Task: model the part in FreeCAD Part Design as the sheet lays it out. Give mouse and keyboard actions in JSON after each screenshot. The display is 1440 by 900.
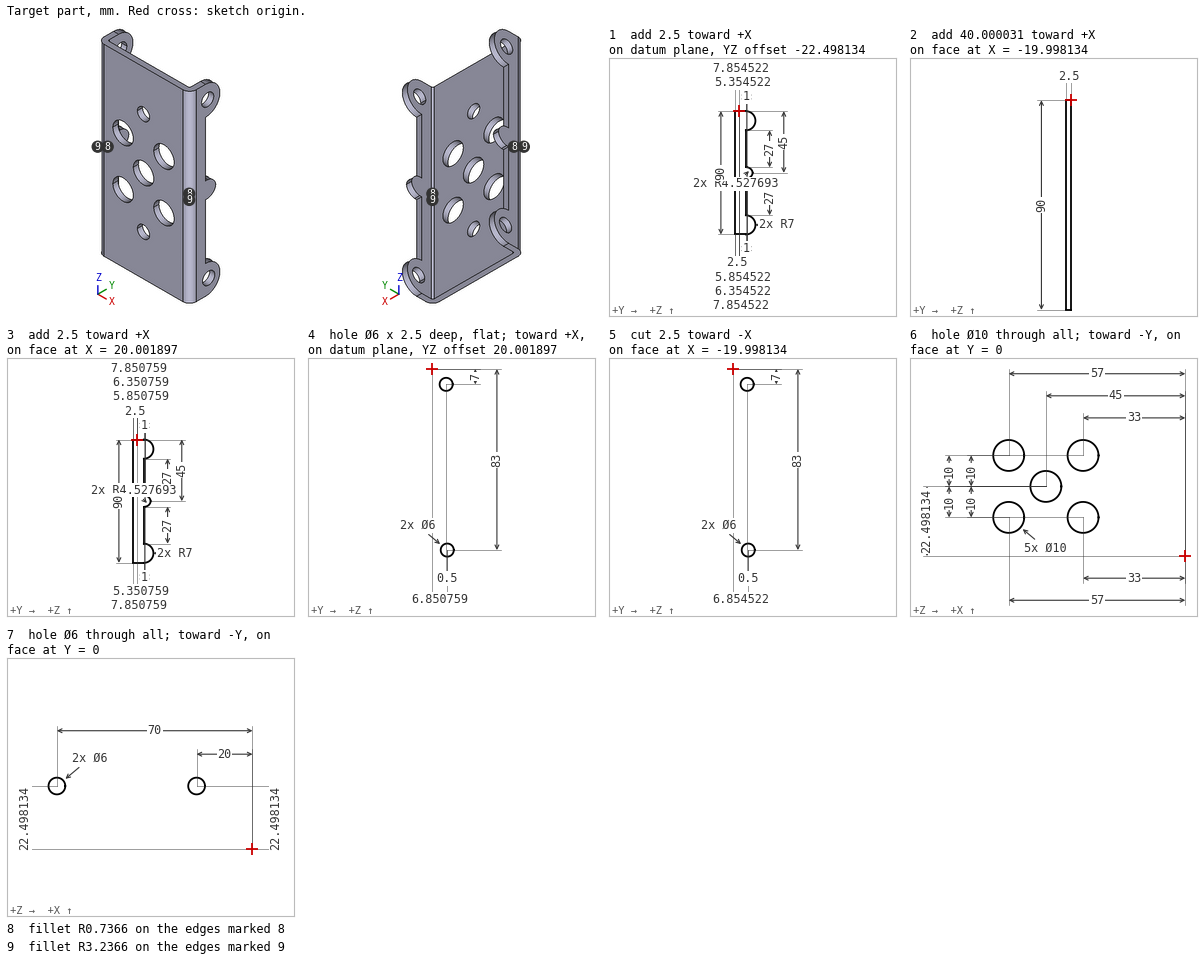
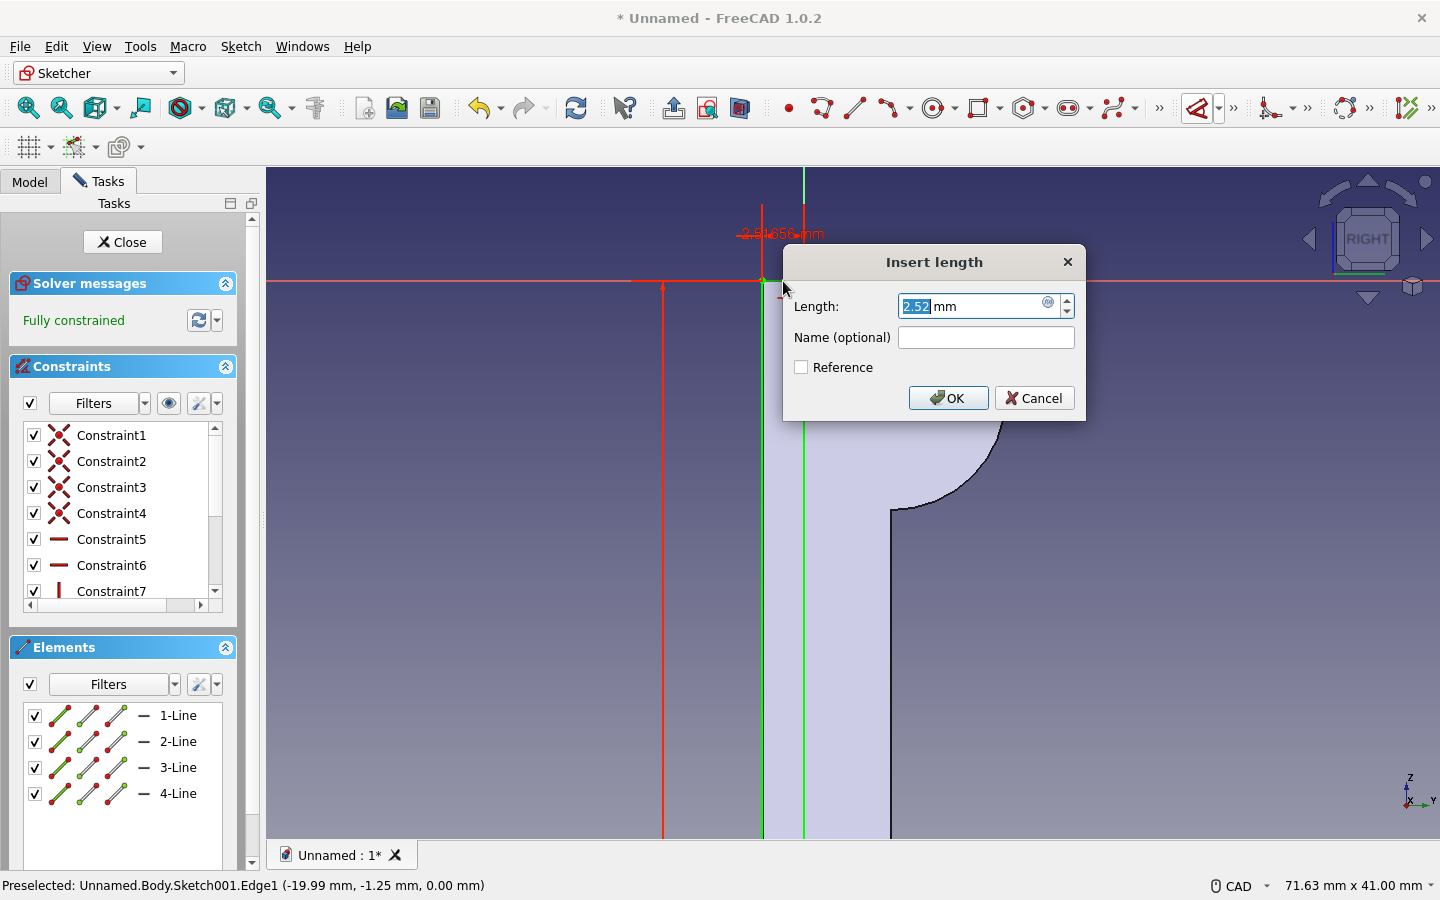
{"action": "type", "text": "2.5"}
{"action": "key", "text": "Return"}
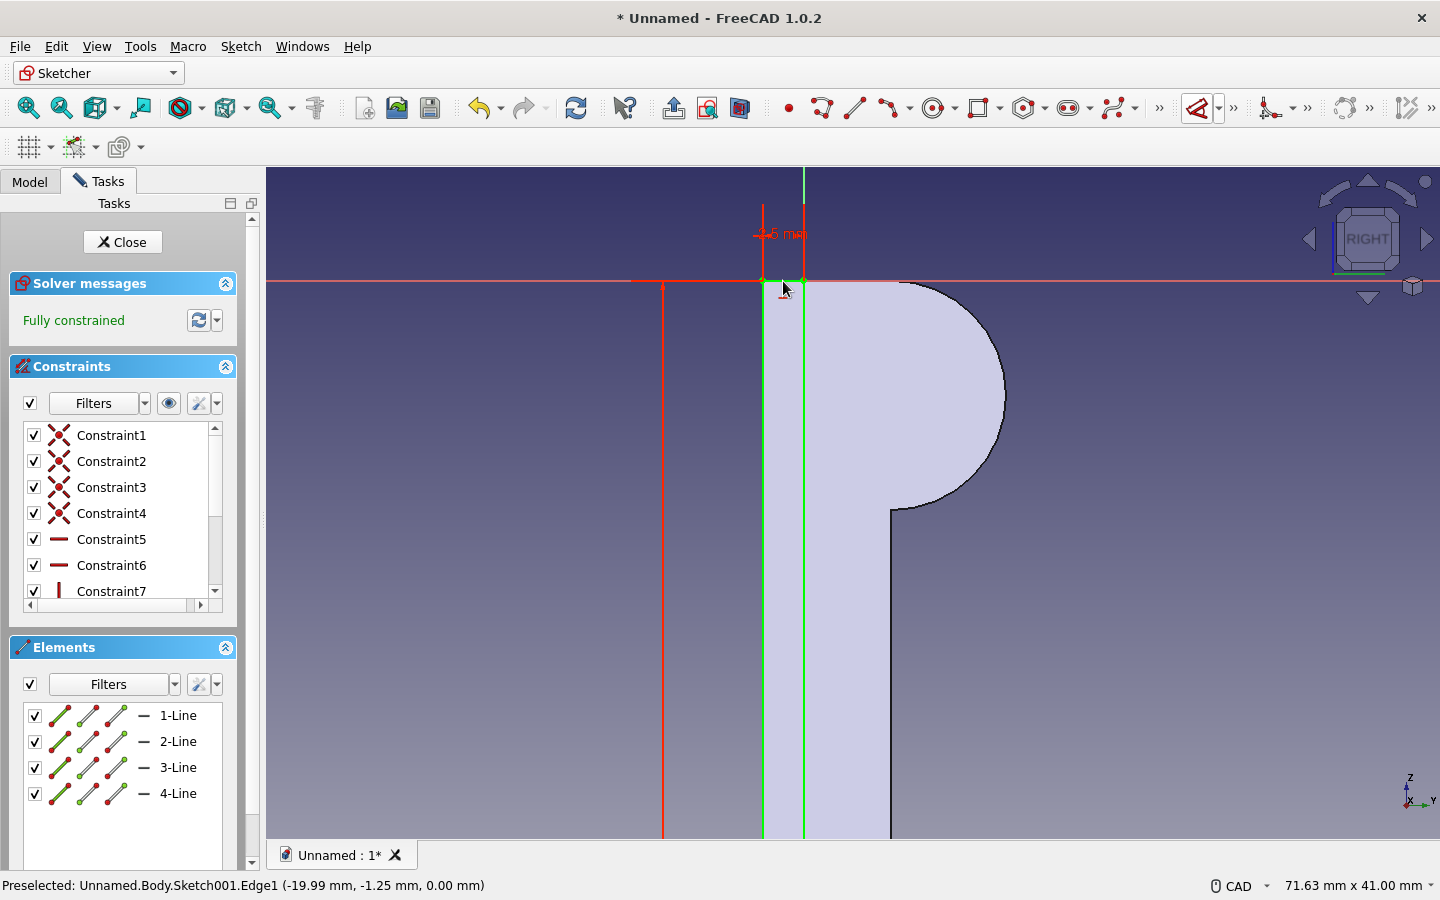
{"action": "left_click", "coordinate": [123, 242]}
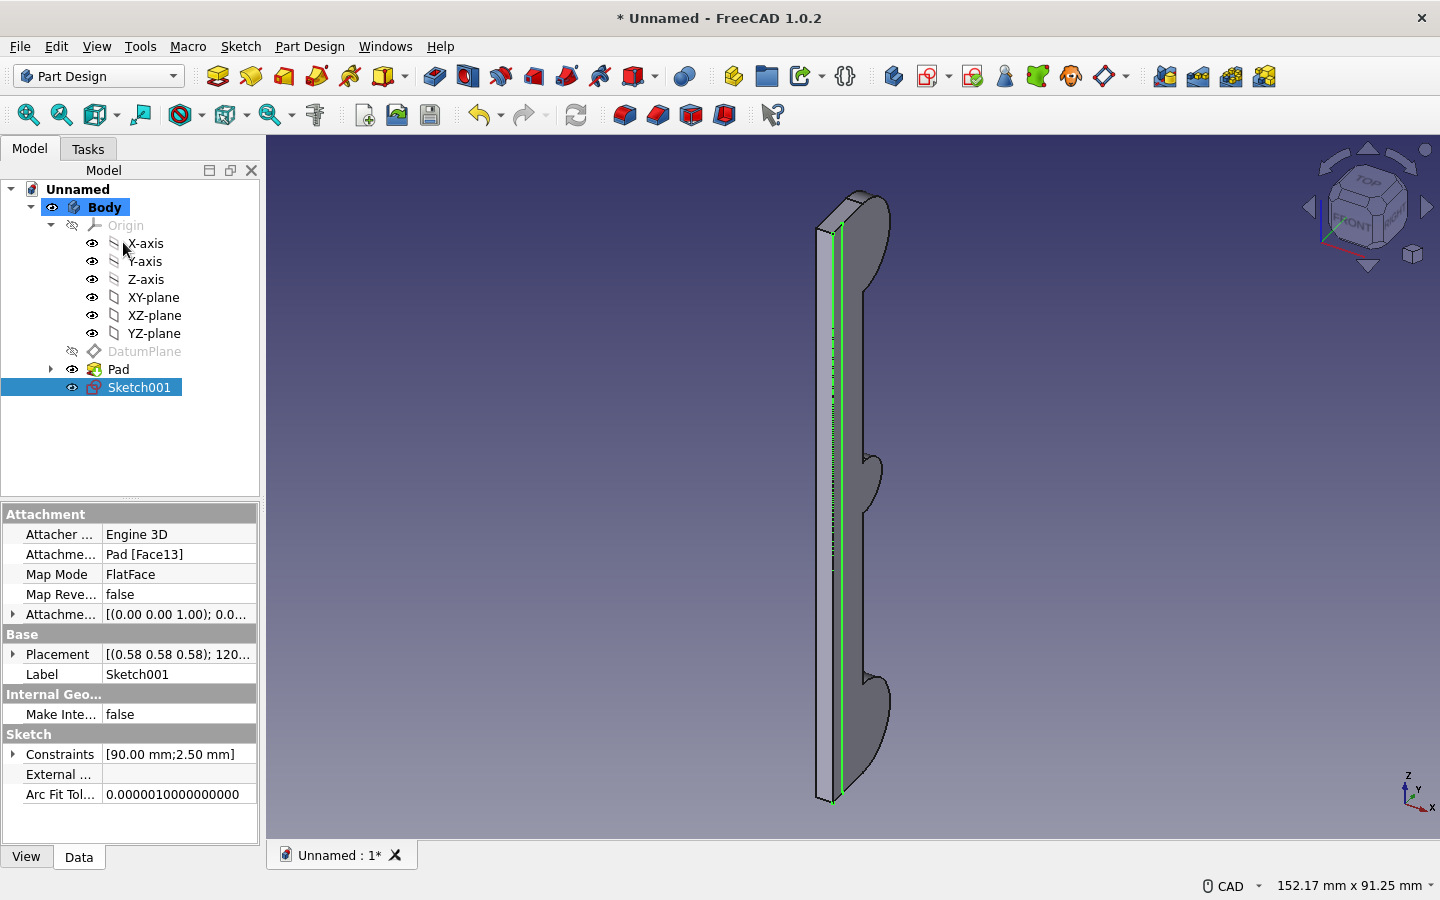
{"action": "left_click", "coordinate": [218, 76]}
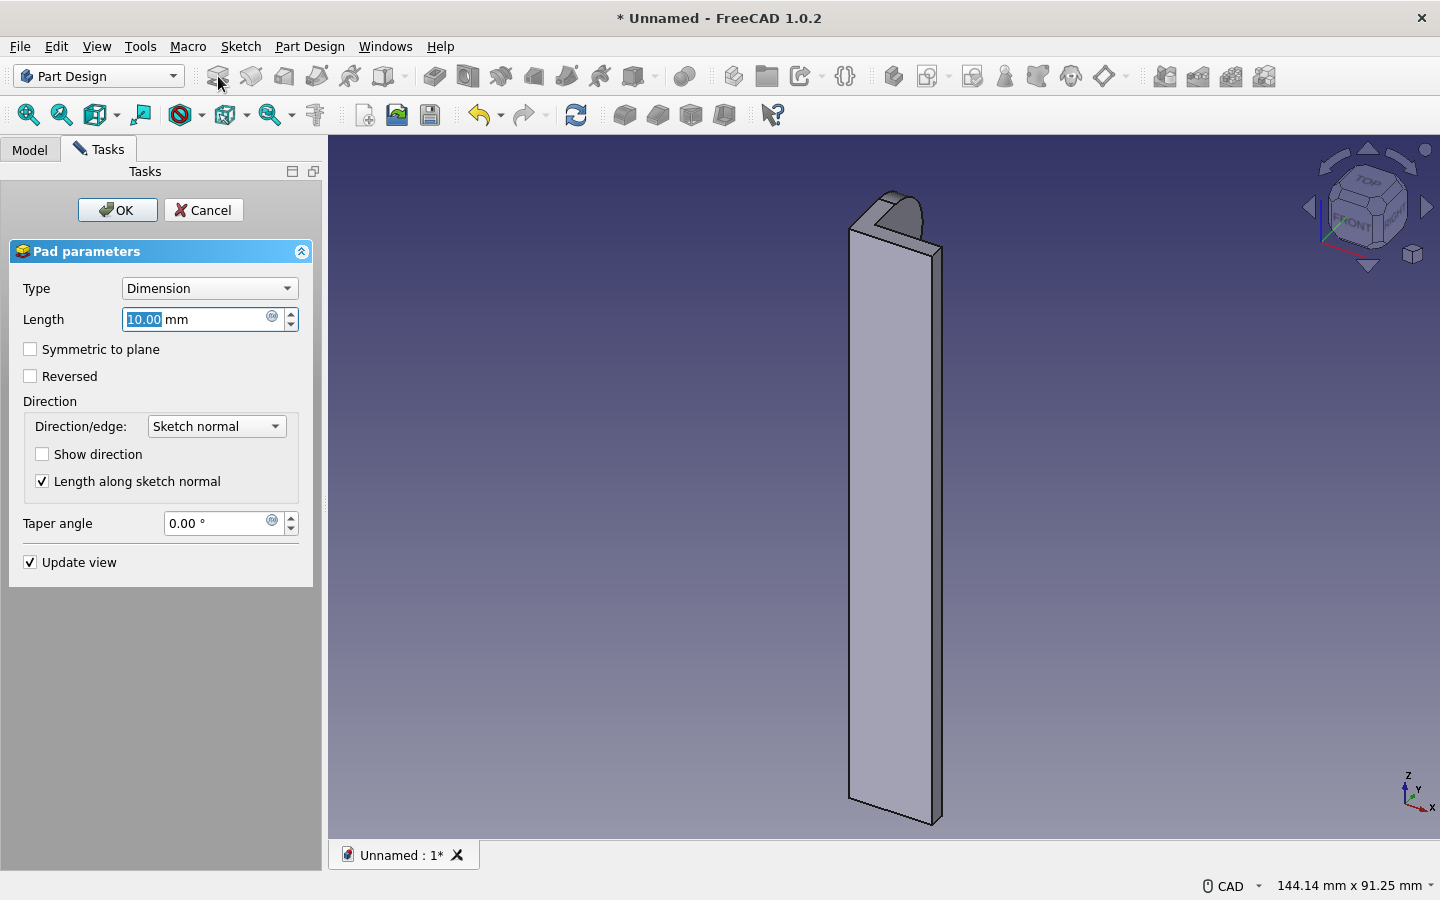
{"action": "type", "text": "40.000031"}
{"action": "key", "text": "Tab"}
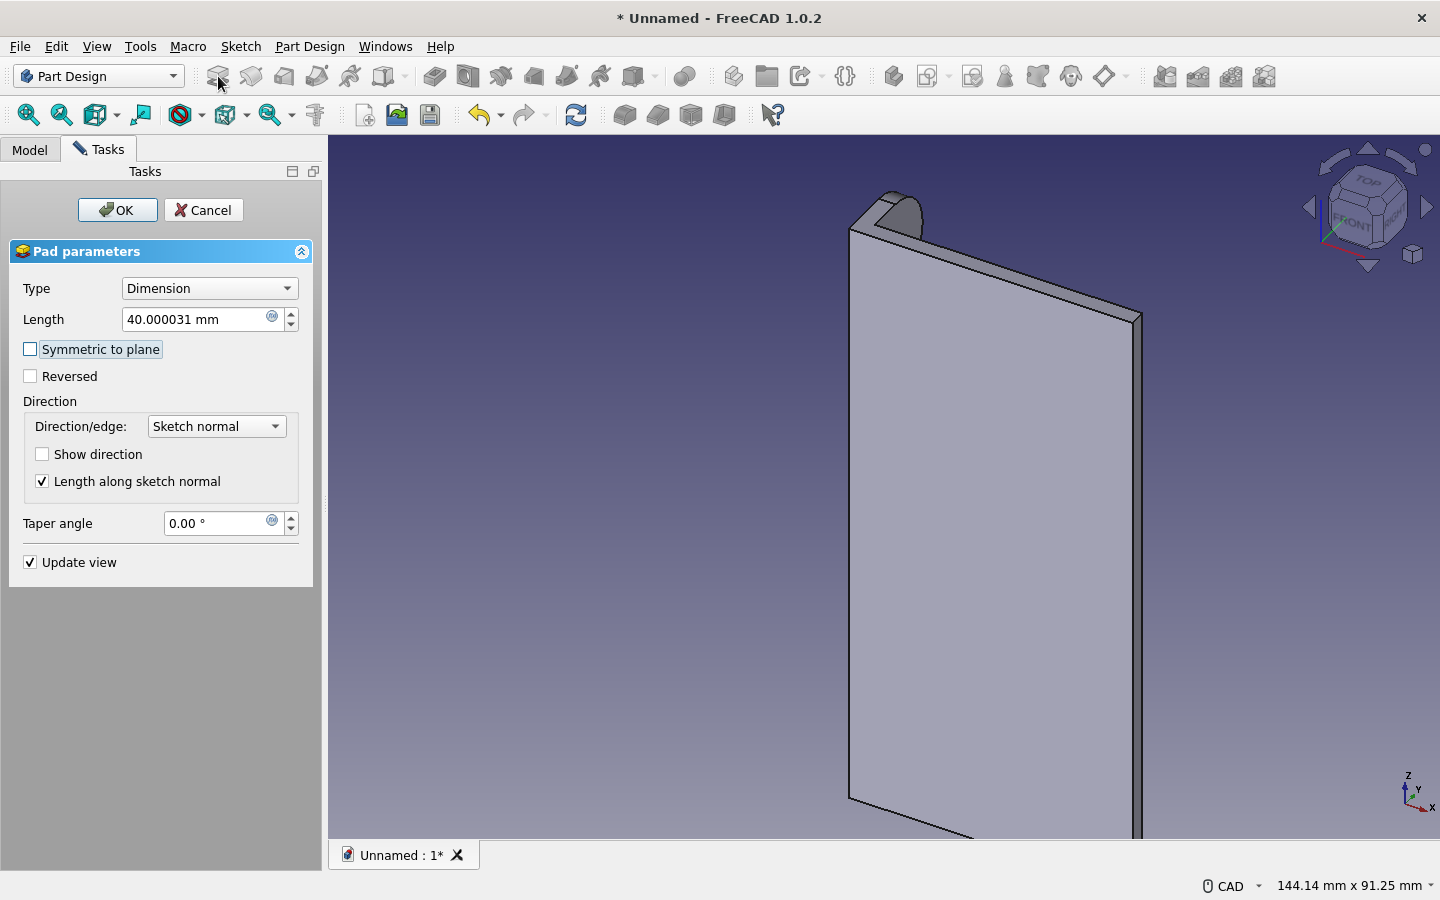
{"action": "left_click", "coordinate": [118, 210]}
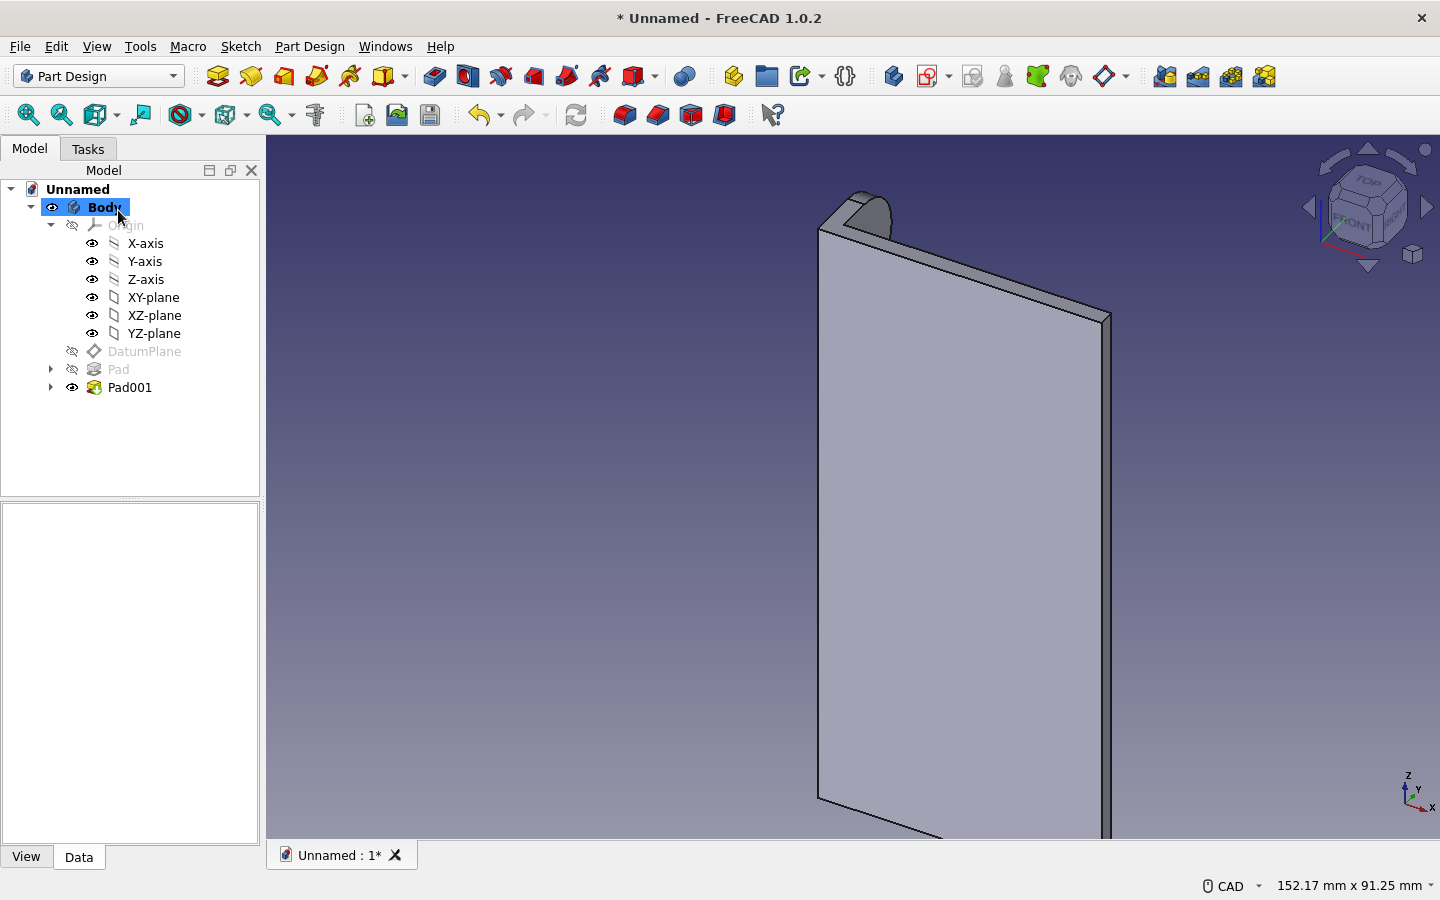
{"action": "left_click", "coordinate": [29, 116]}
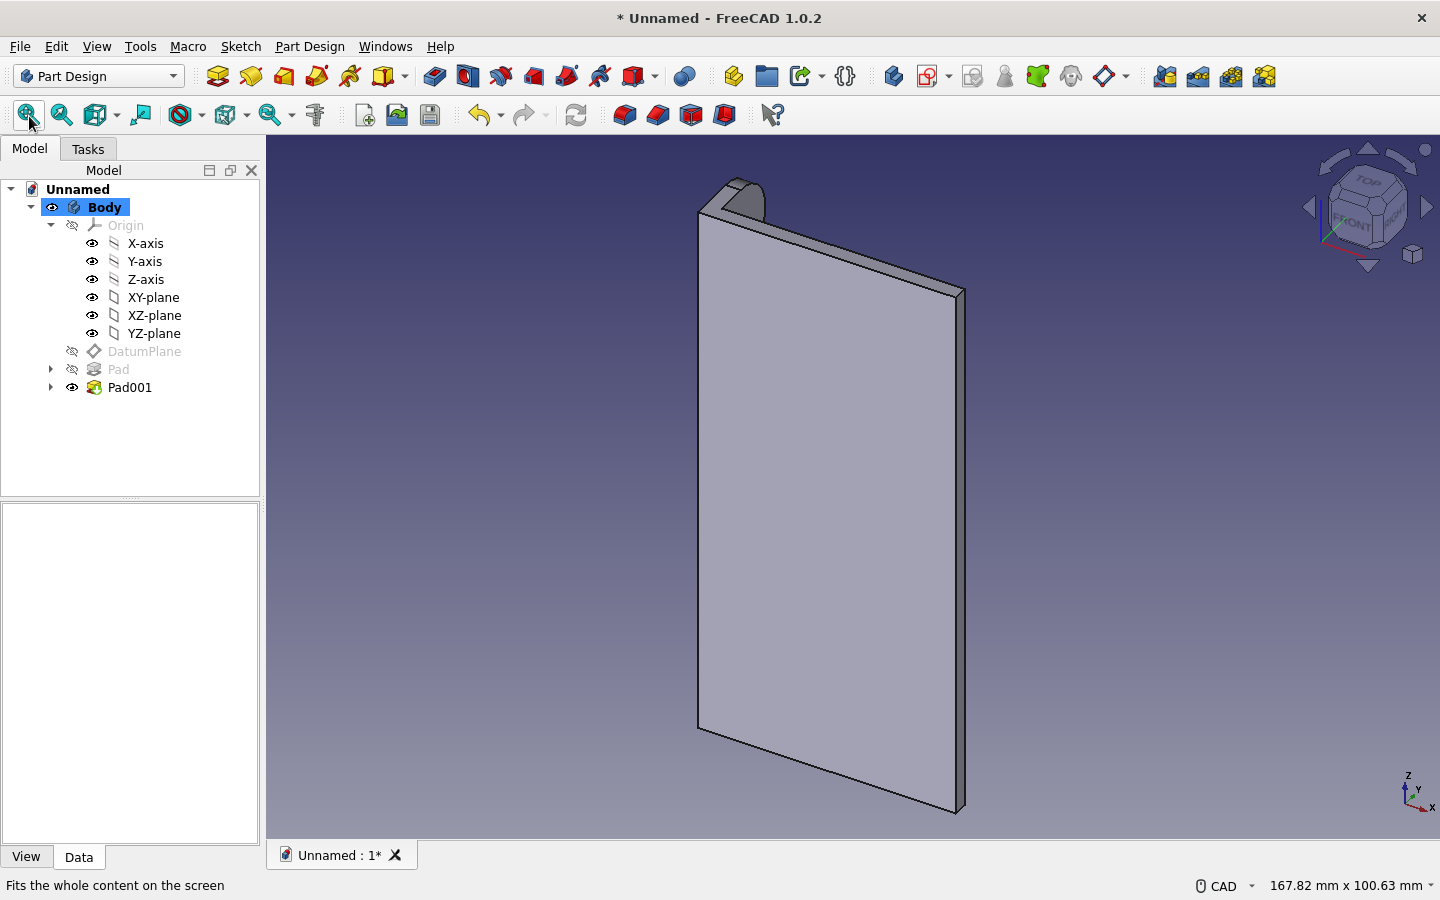
{"action": "key", "text": "0"}